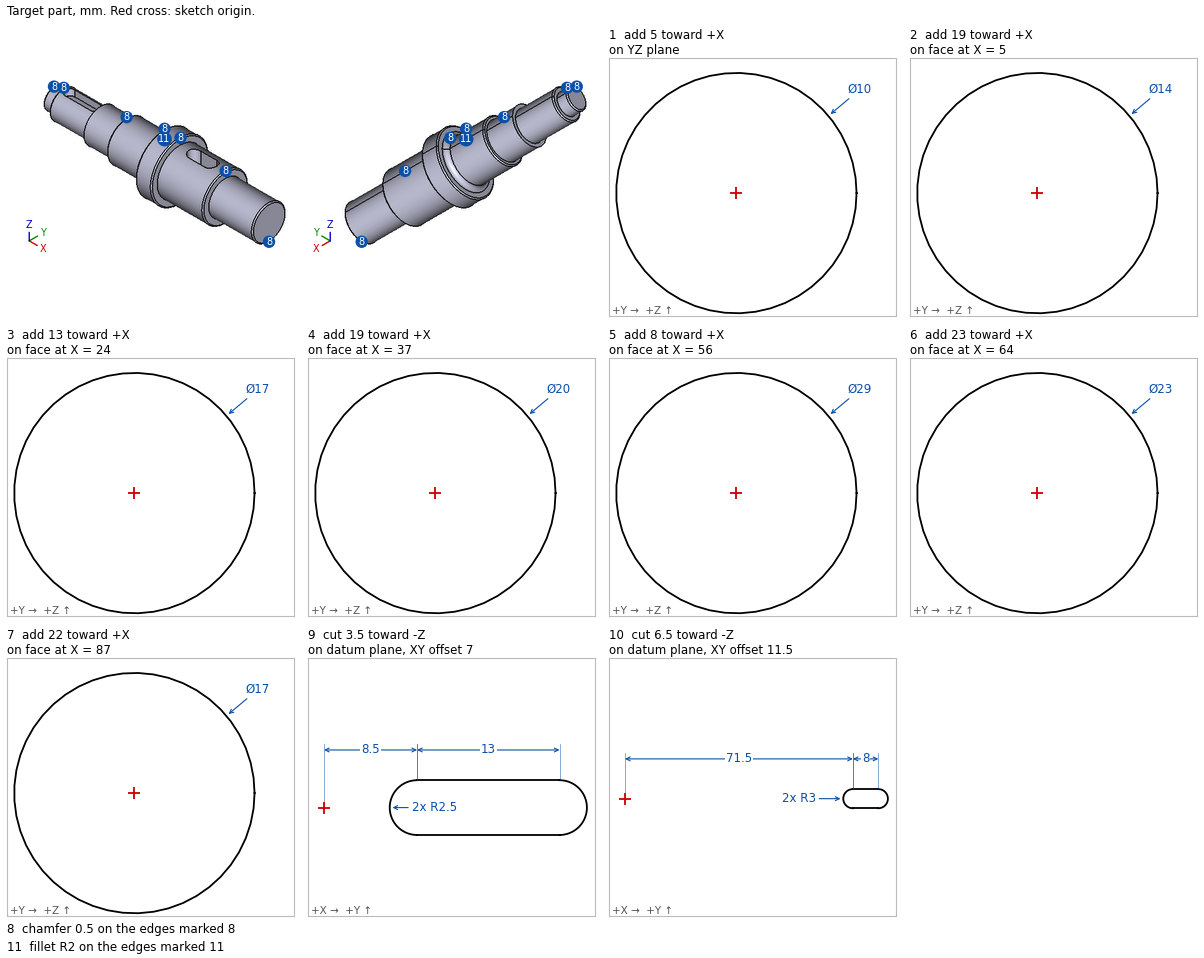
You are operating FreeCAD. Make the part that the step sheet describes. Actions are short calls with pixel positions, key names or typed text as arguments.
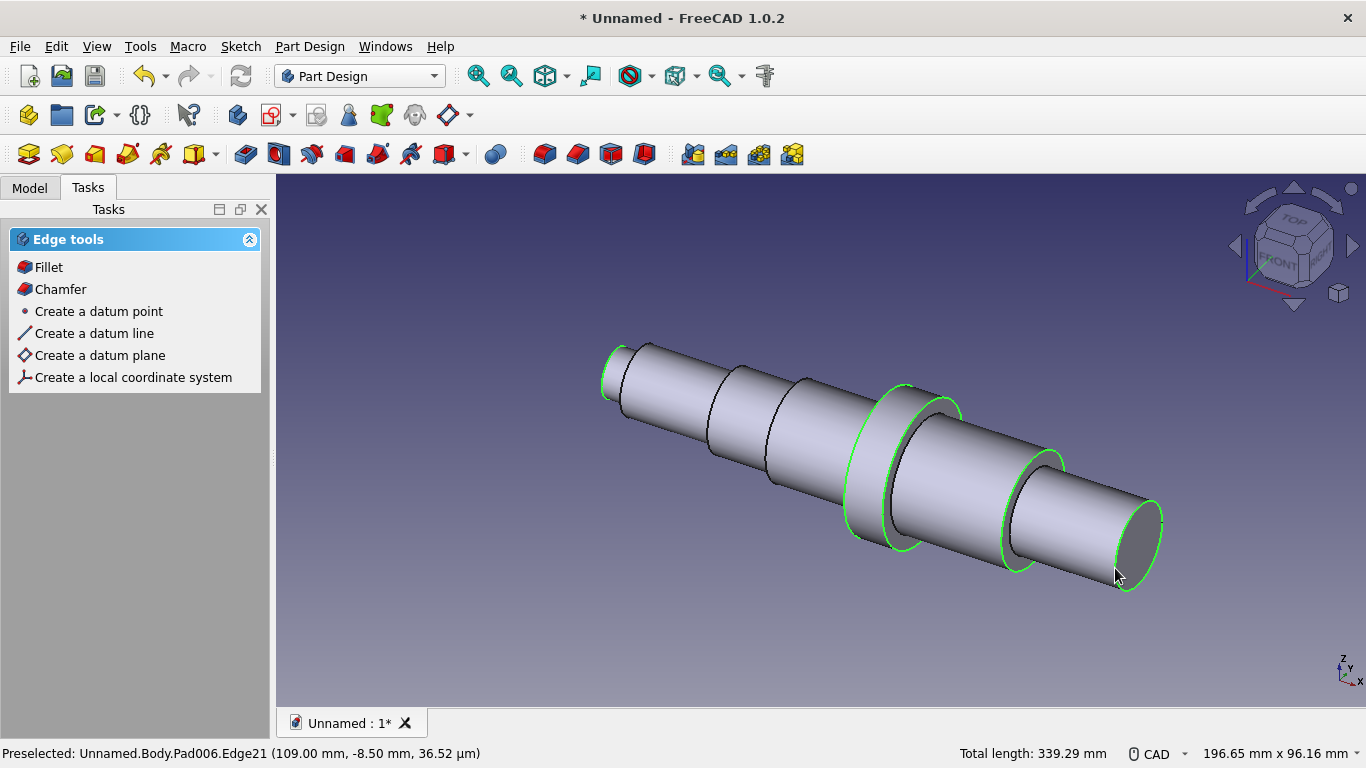
click(624, 414, ctrl)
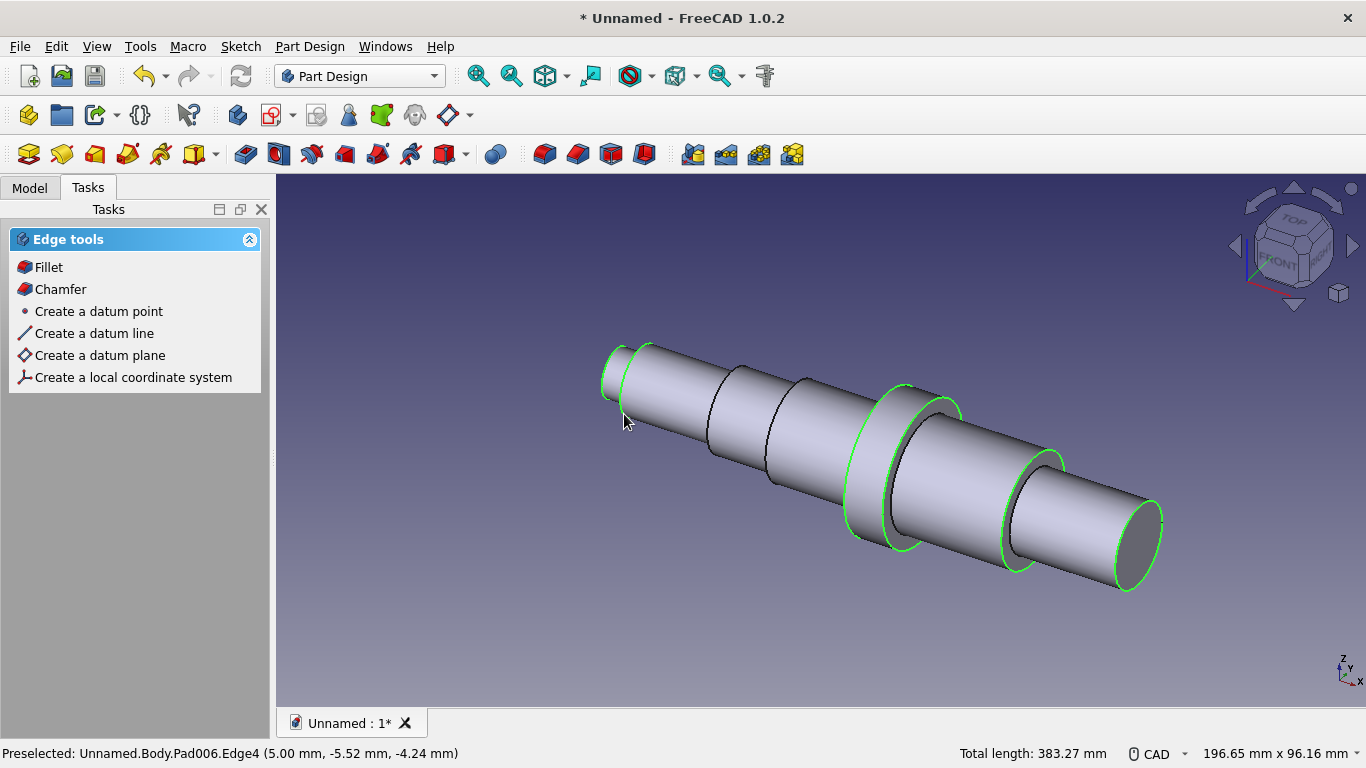
key(0)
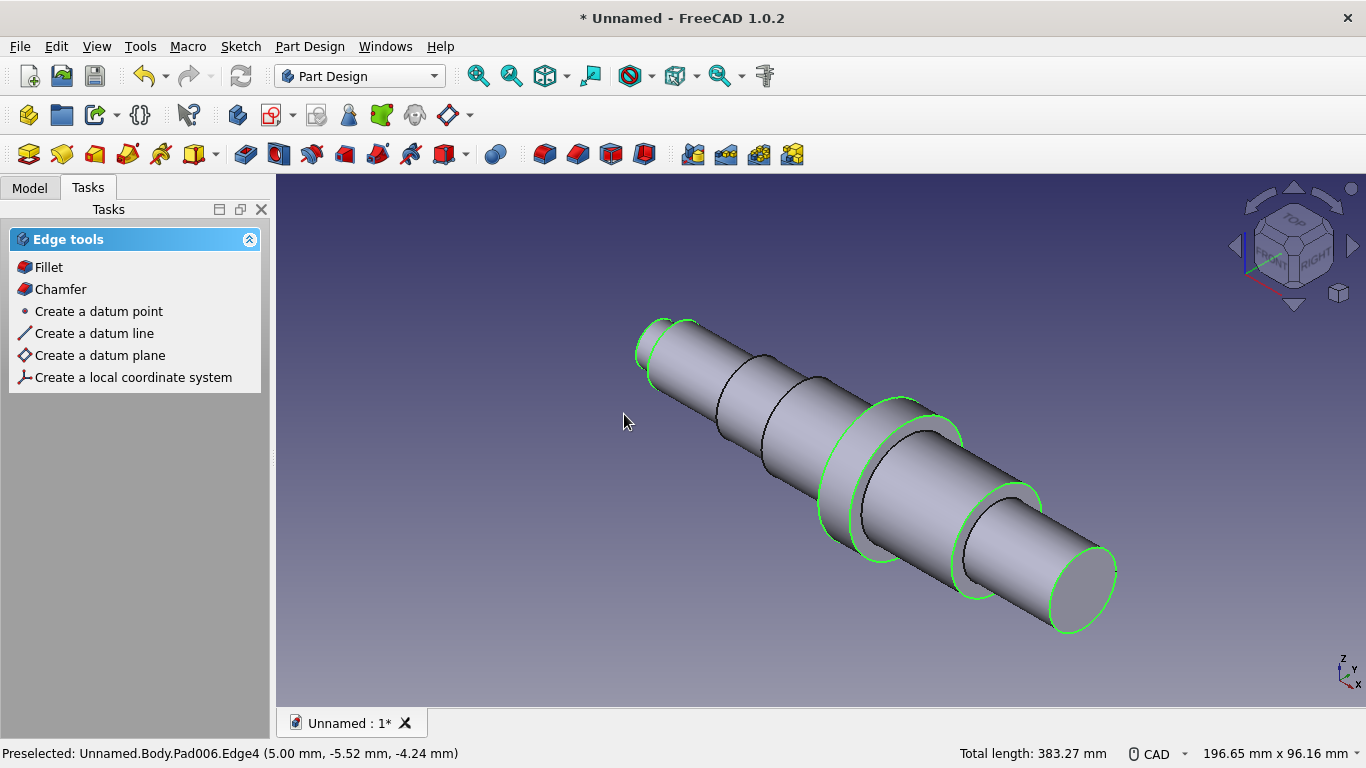
key(2)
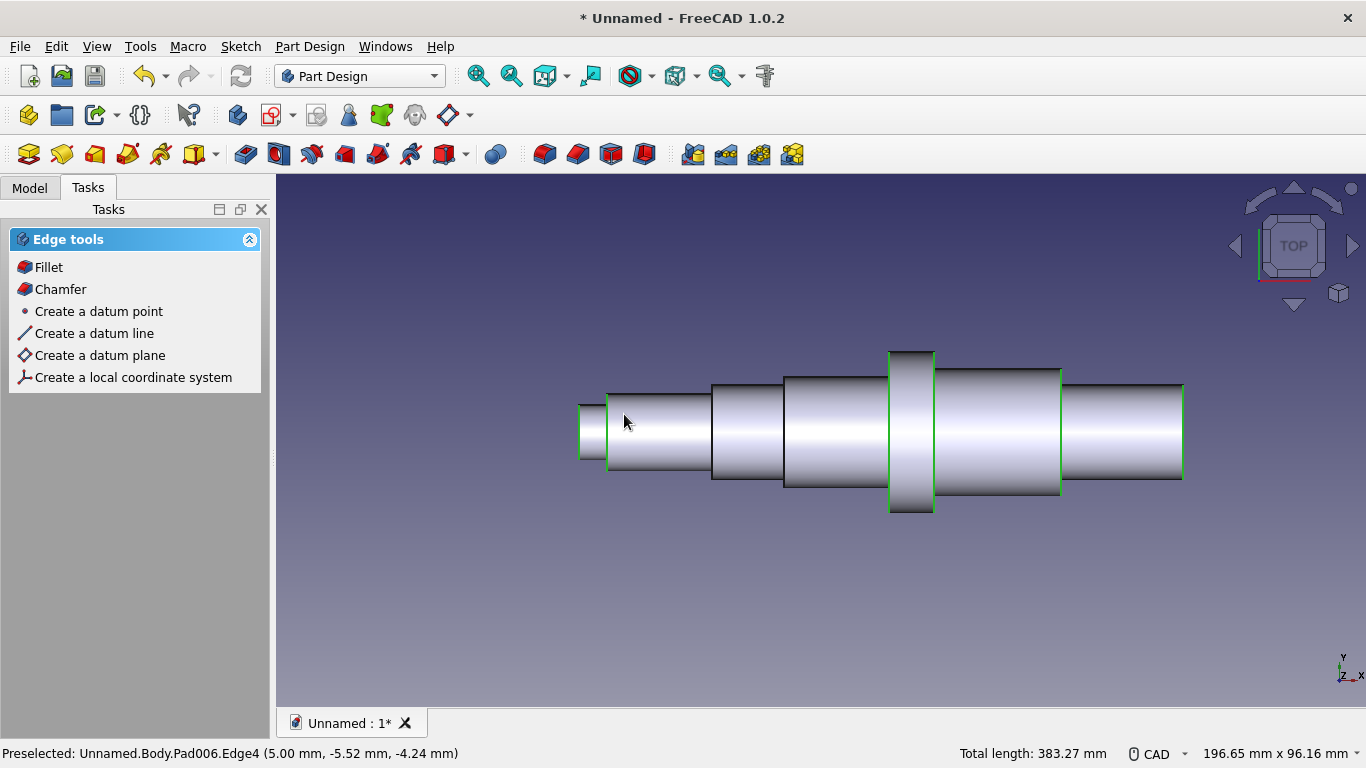
click(784, 476, ctrl)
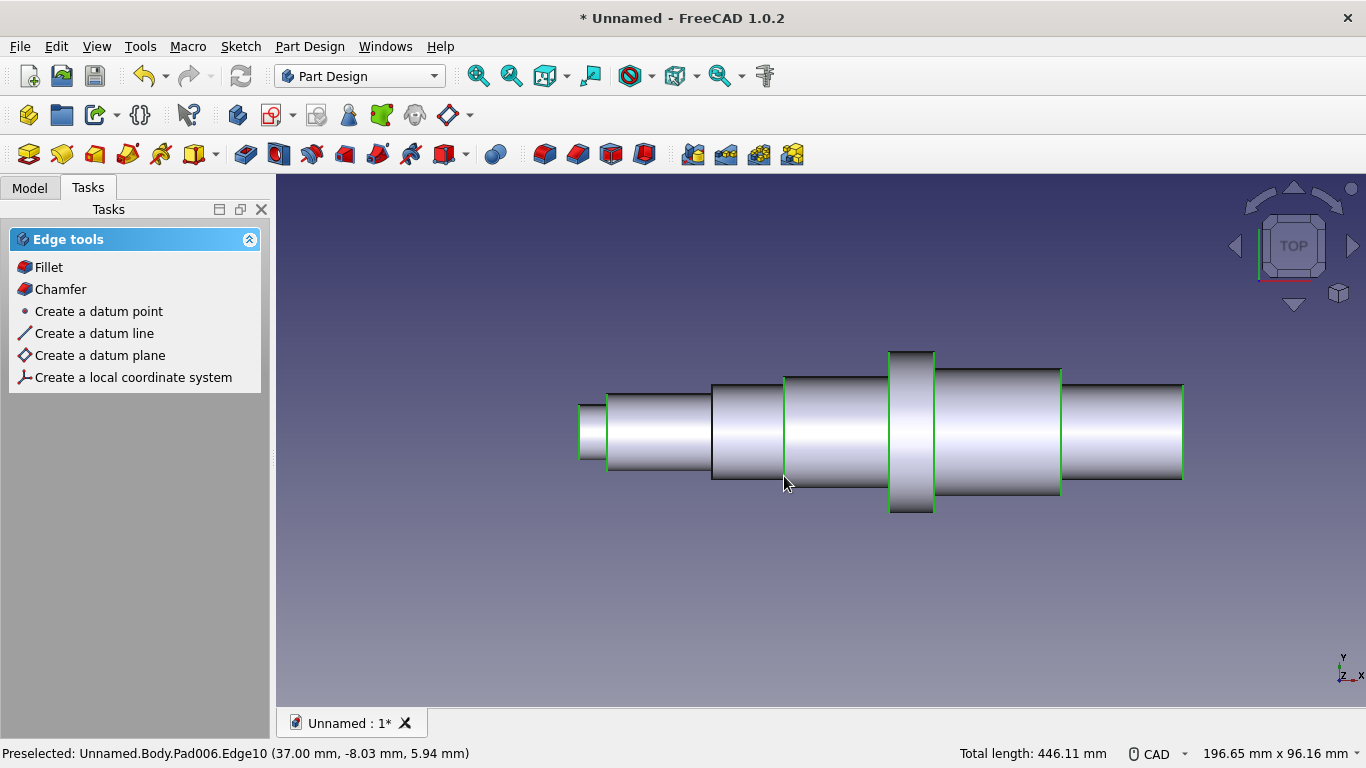
click(578, 154)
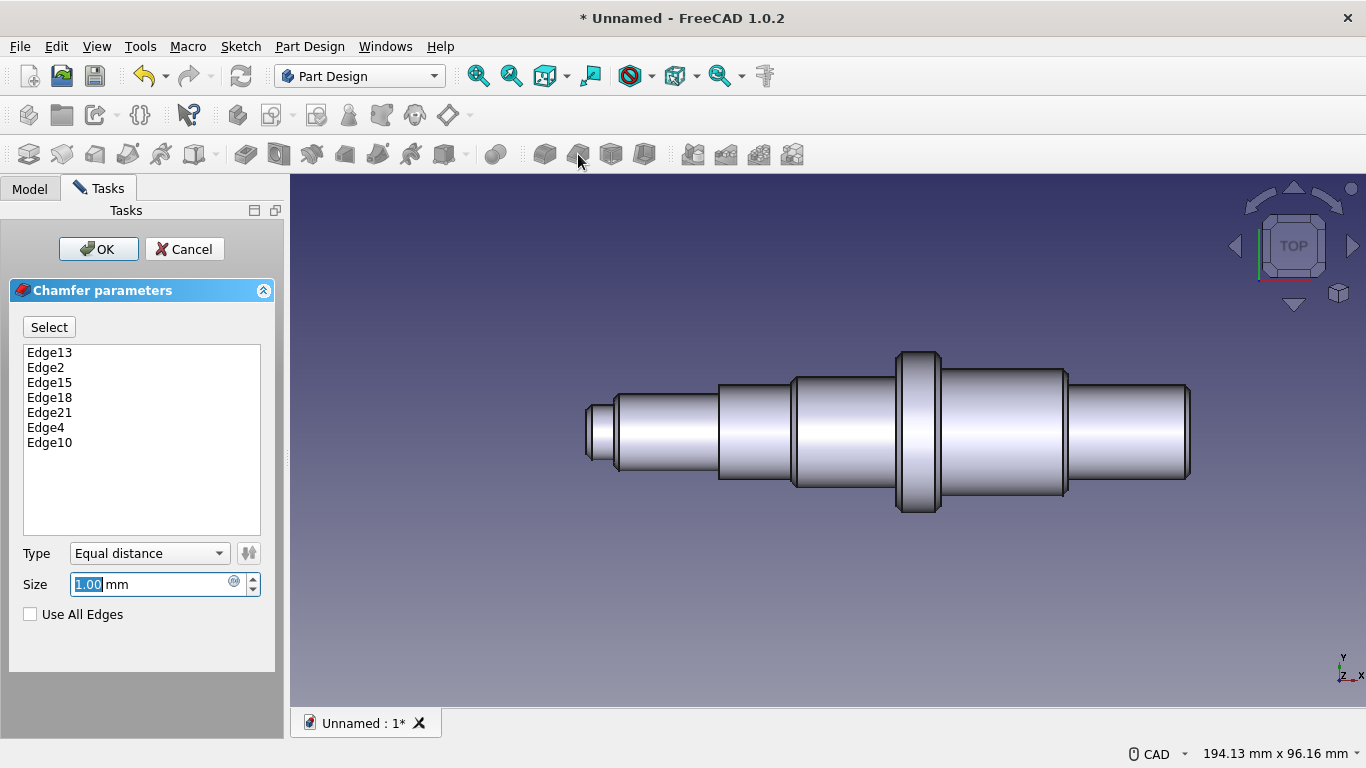
text(0.5)
key(Tab)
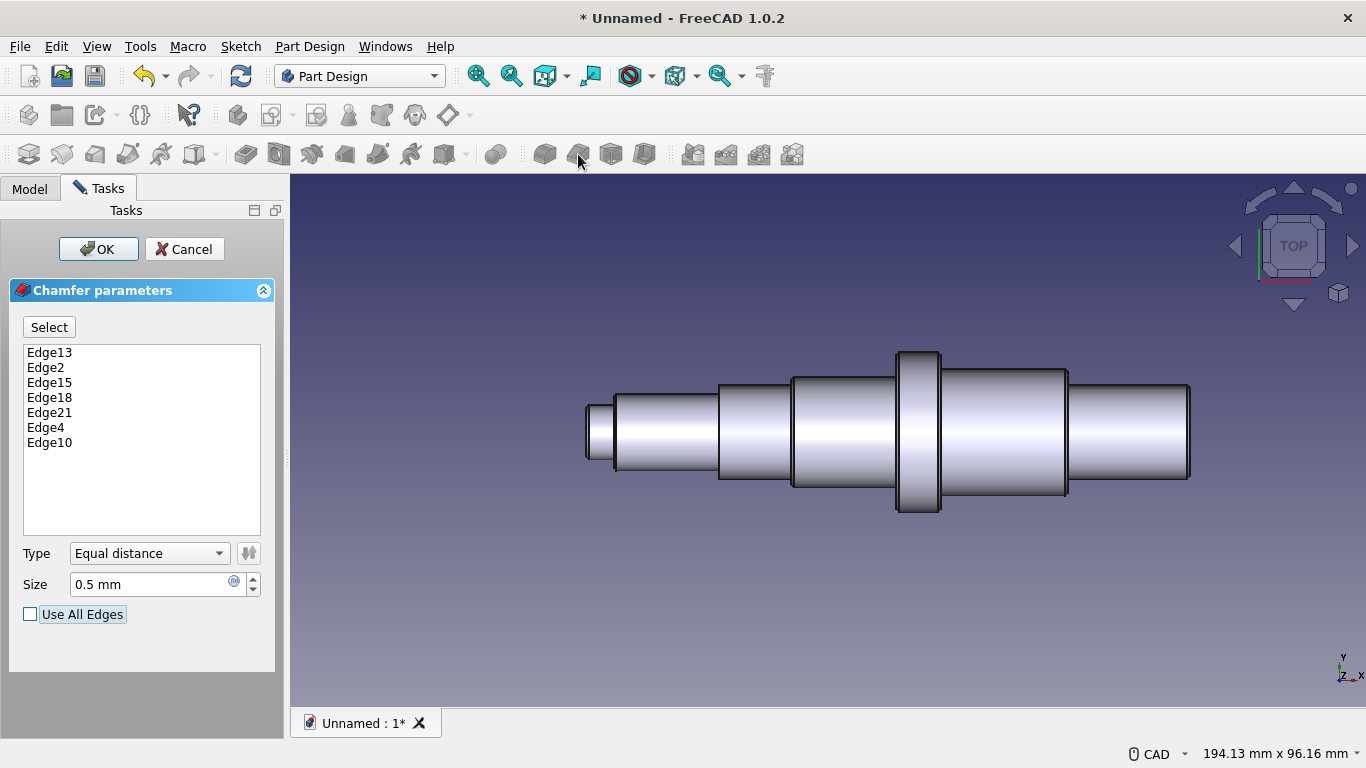
click(99, 249)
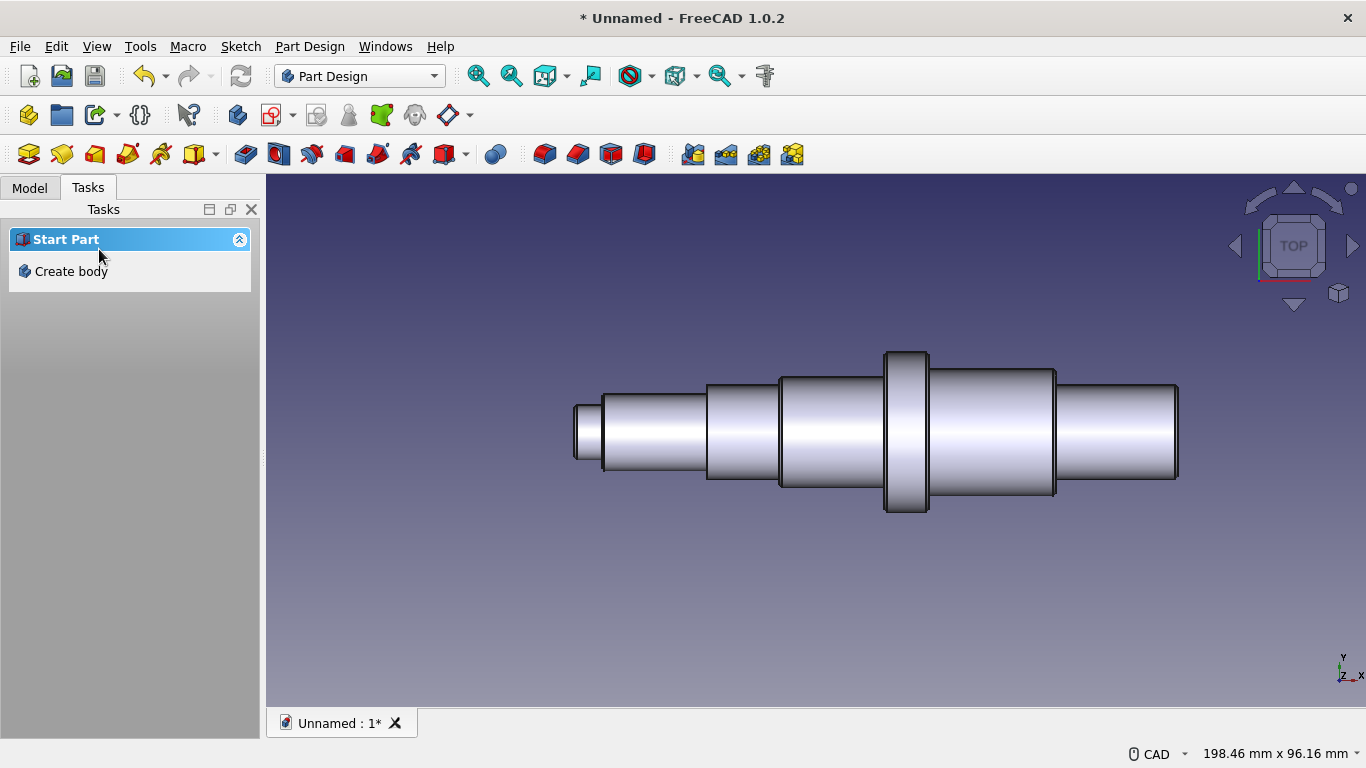
click(30, 188)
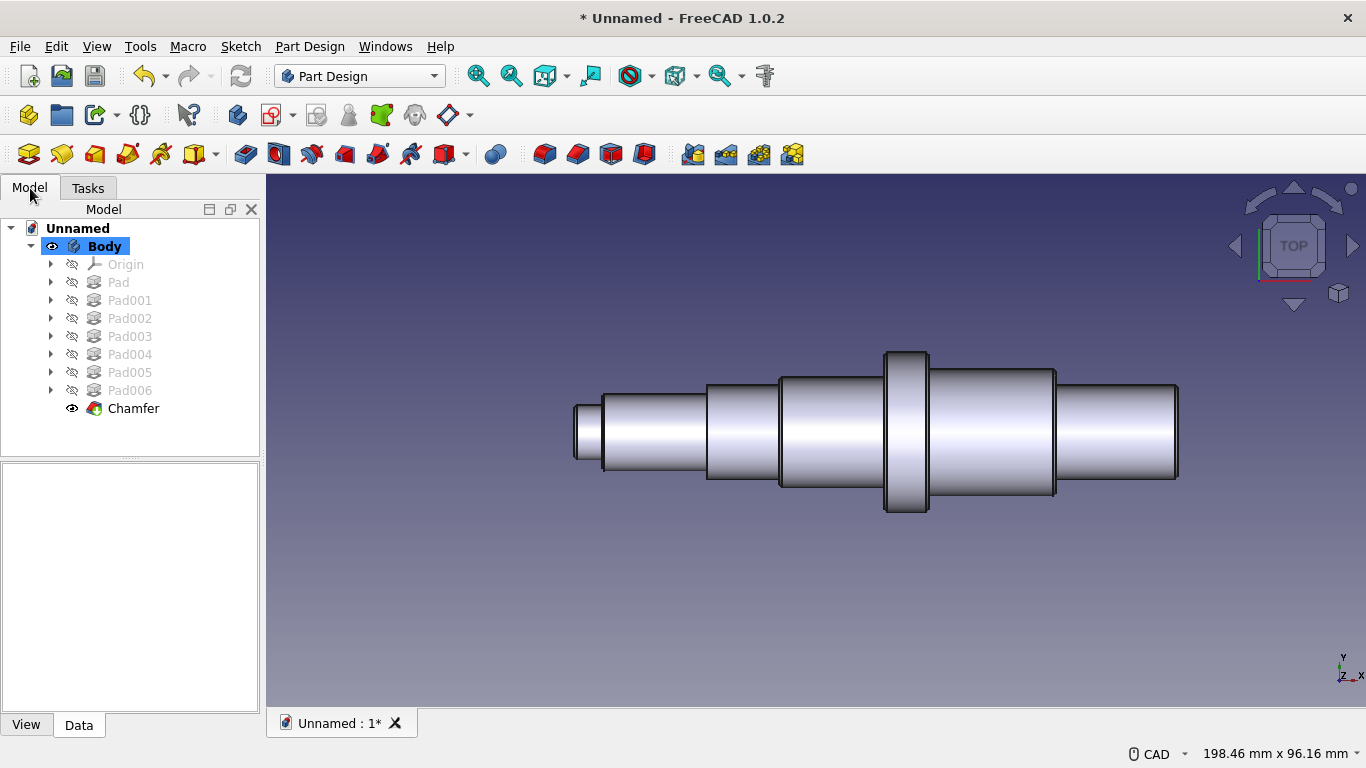
click(51, 264)